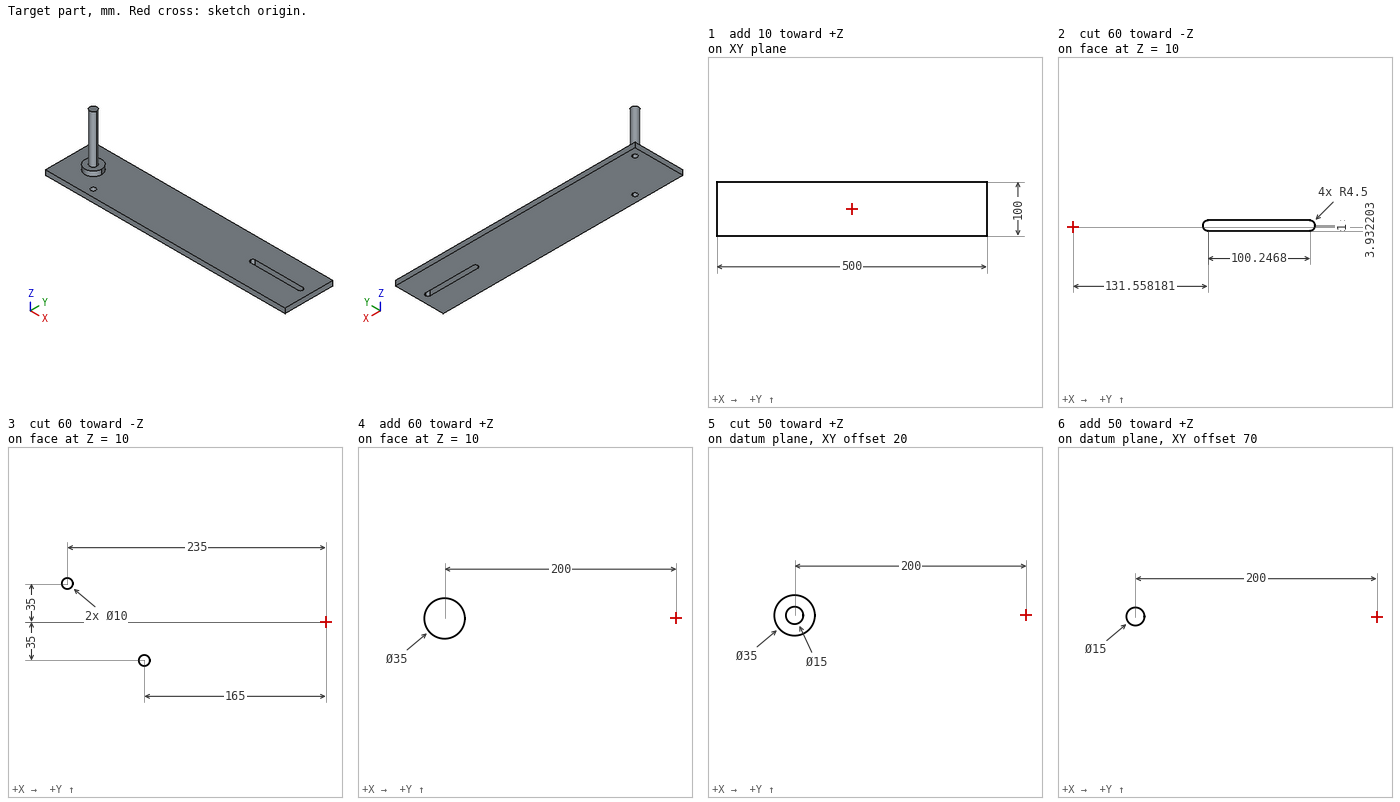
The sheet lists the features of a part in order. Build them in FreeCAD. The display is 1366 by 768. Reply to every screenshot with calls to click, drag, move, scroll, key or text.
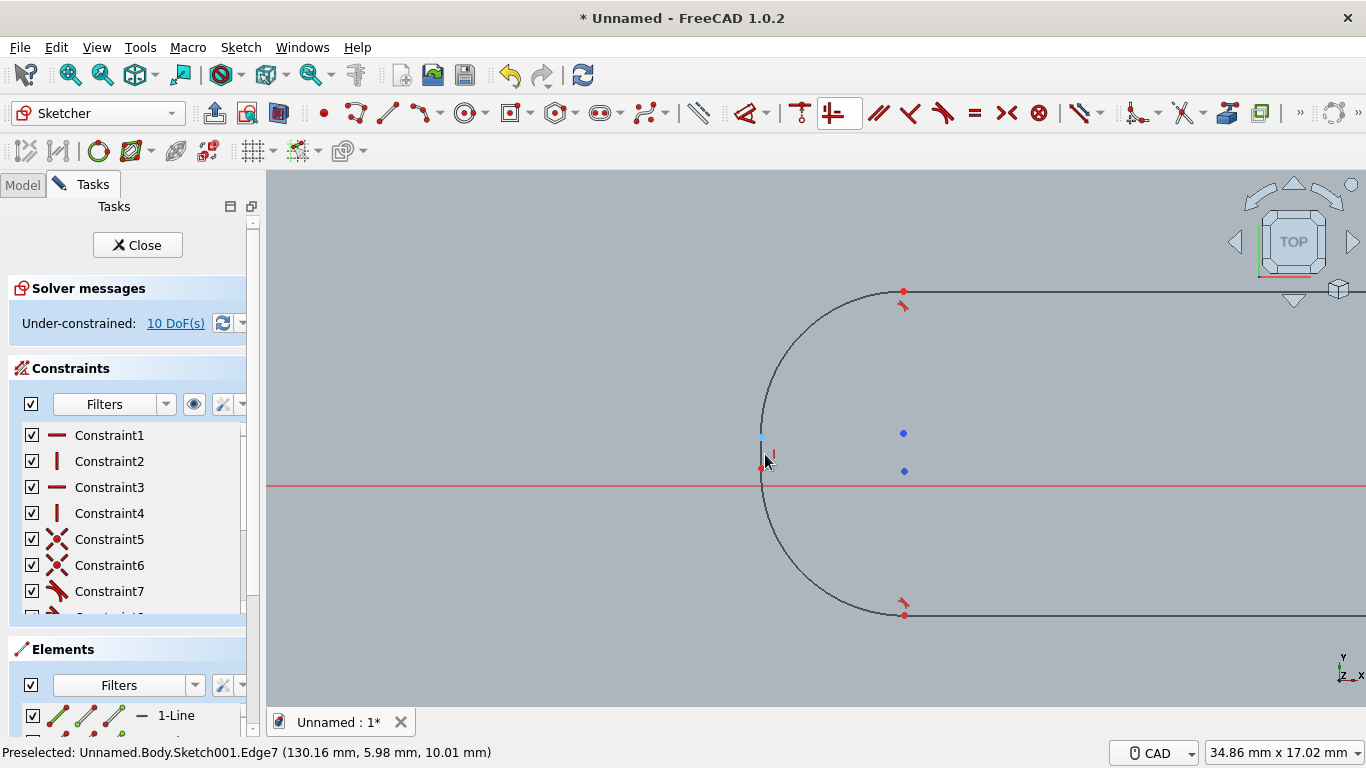
click(761, 453)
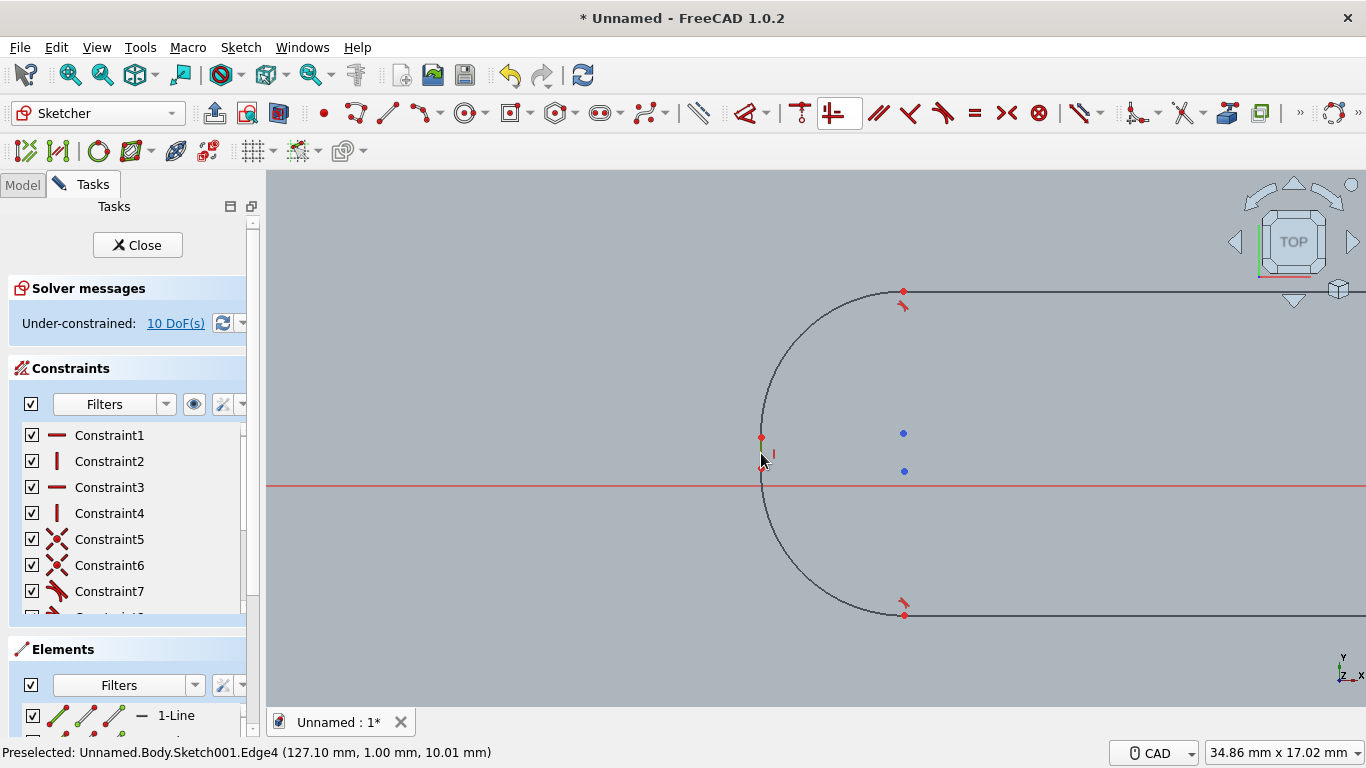
scroll(774, 437, down, 12)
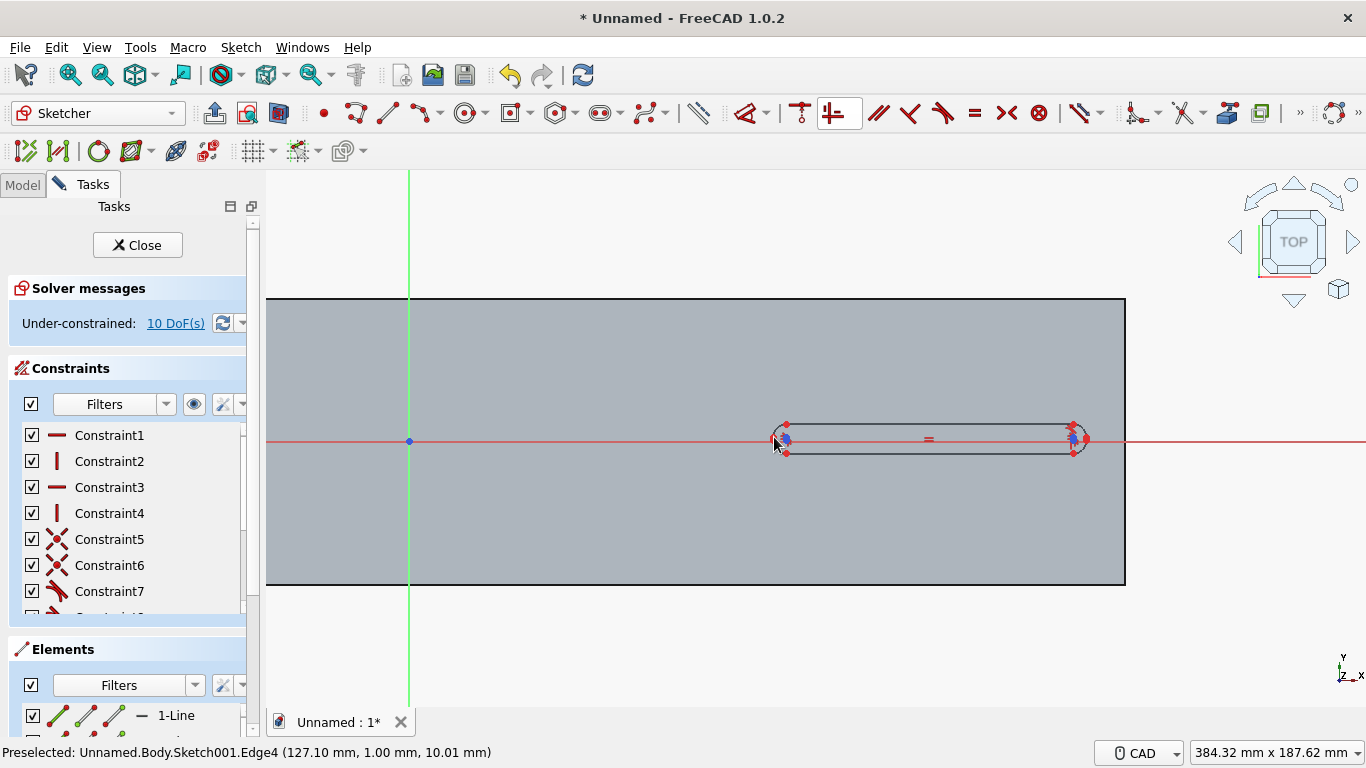
scroll(780, 426, up, 5)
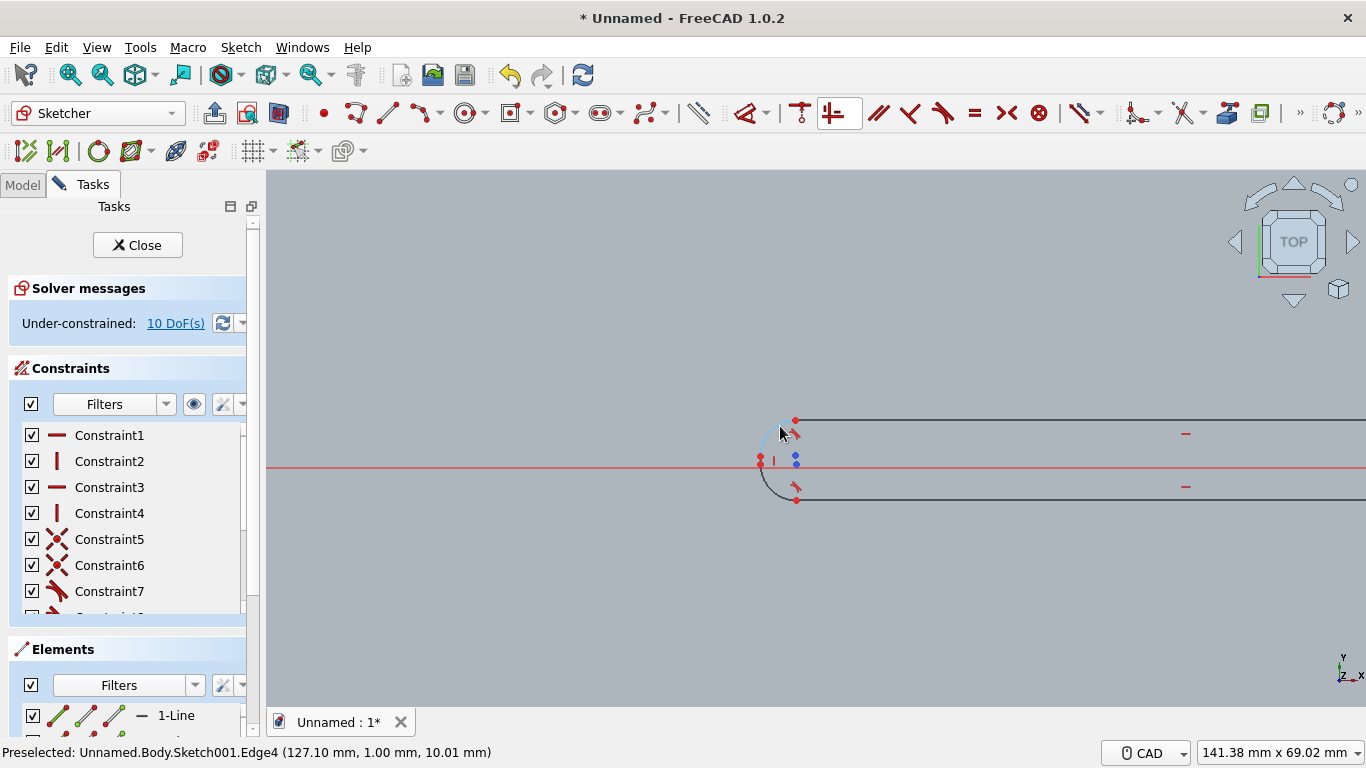
click(780, 424)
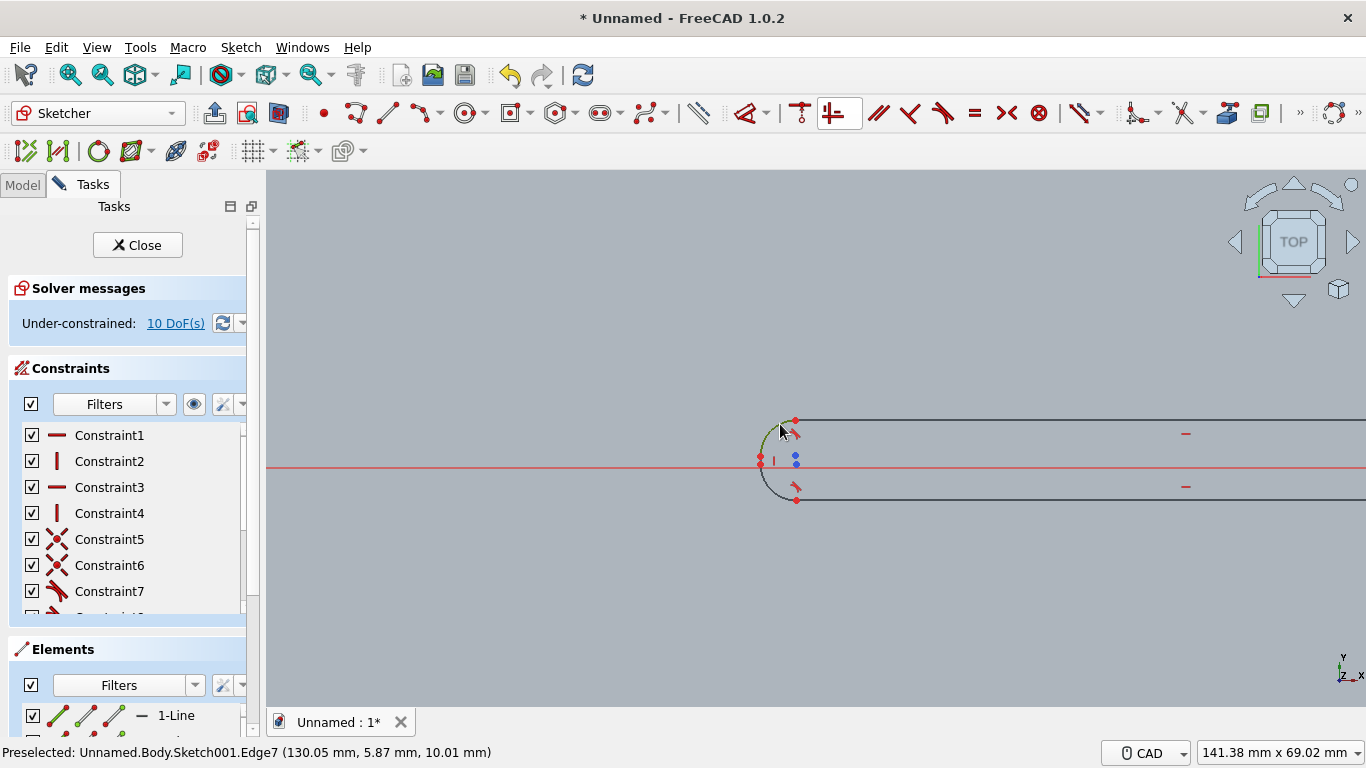
key(t)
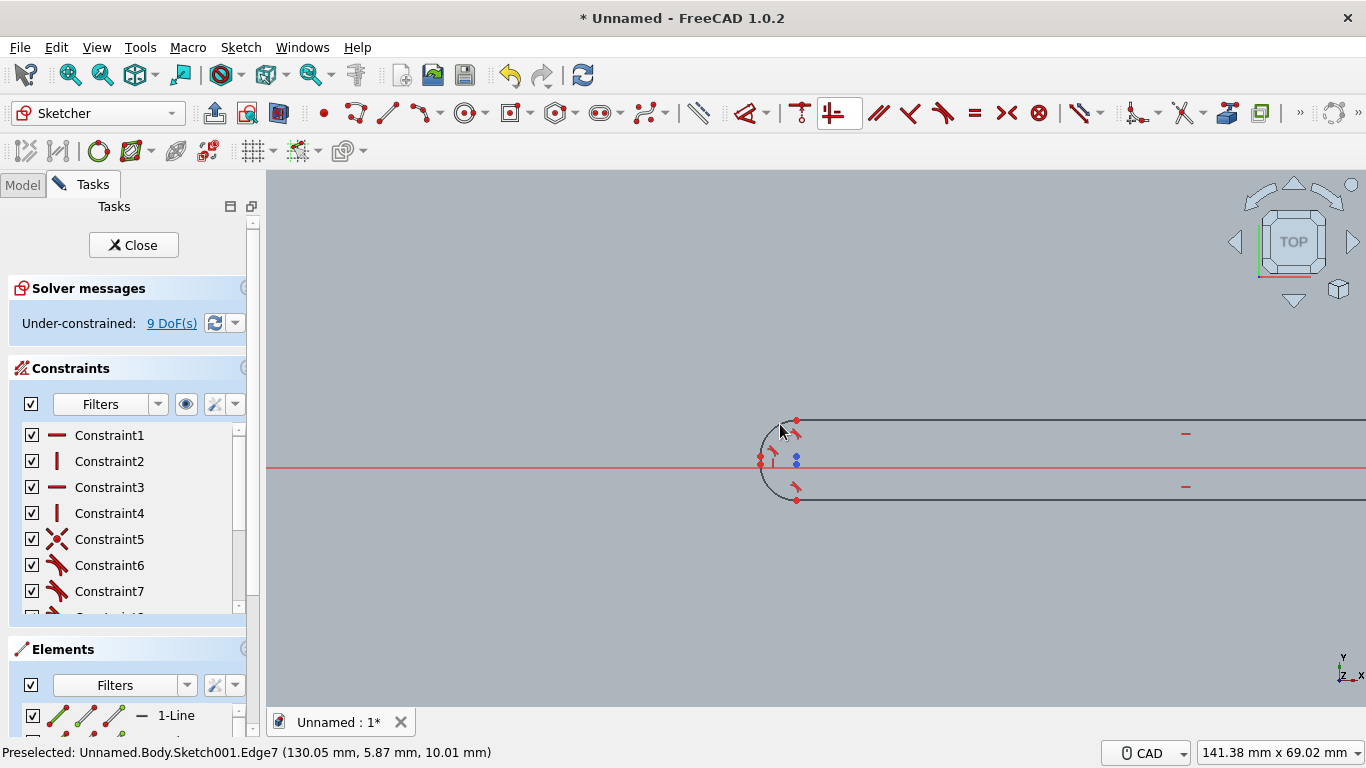
scroll(761, 460, up, 7)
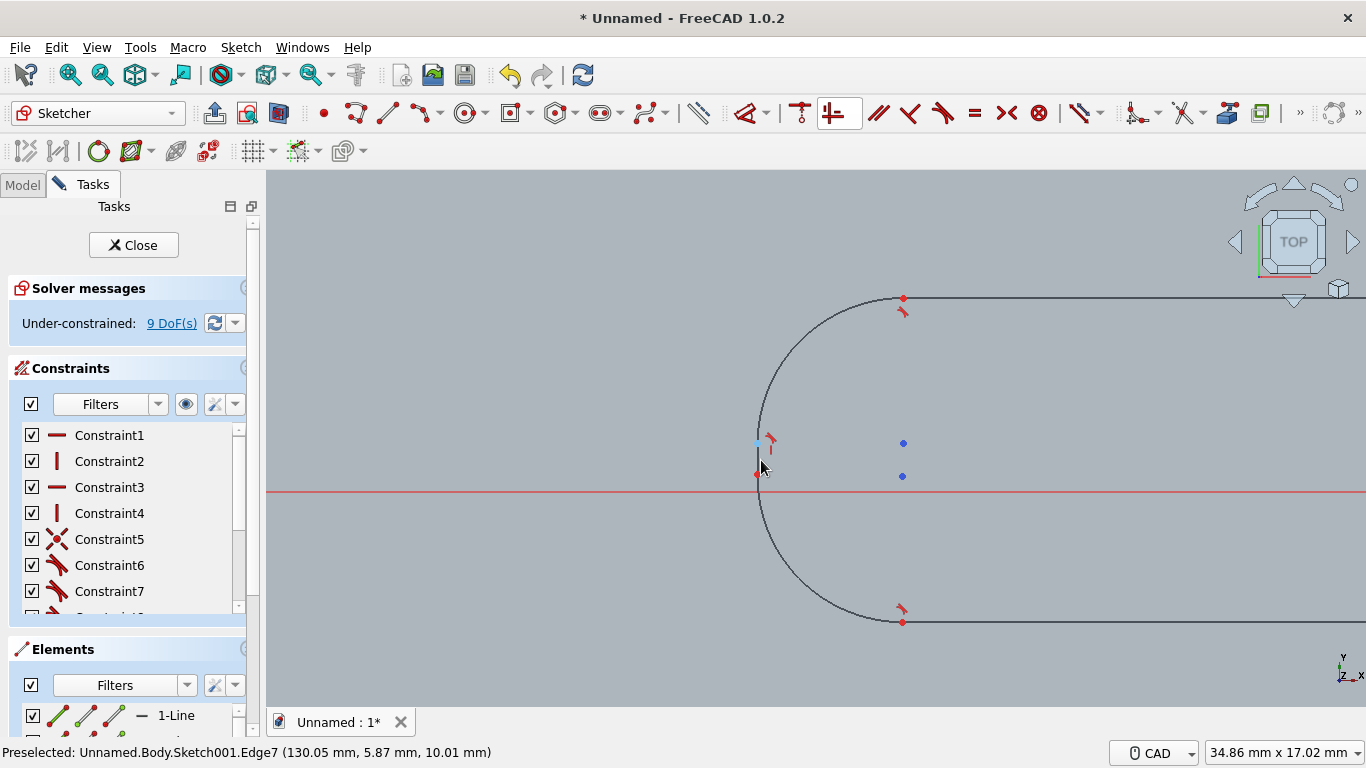
click(758, 459)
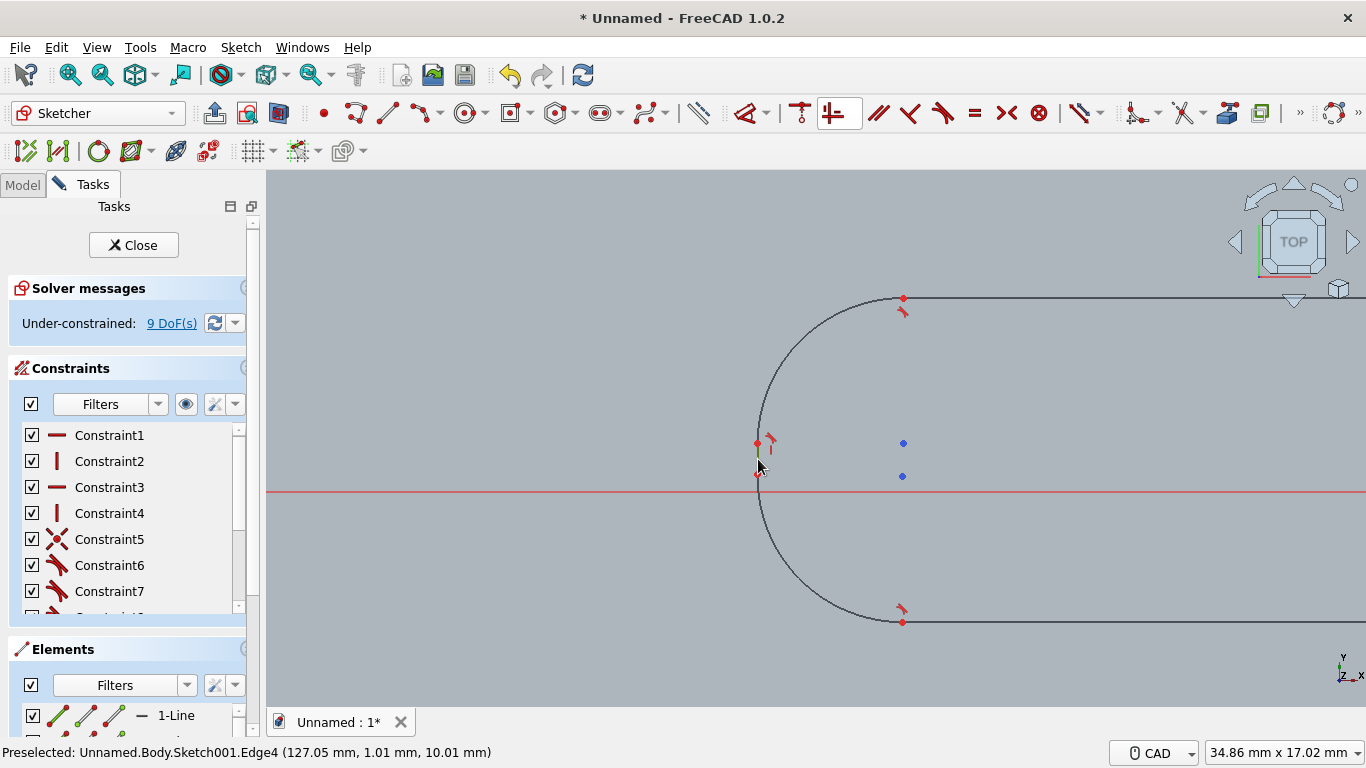
scroll(775, 437, down, 12)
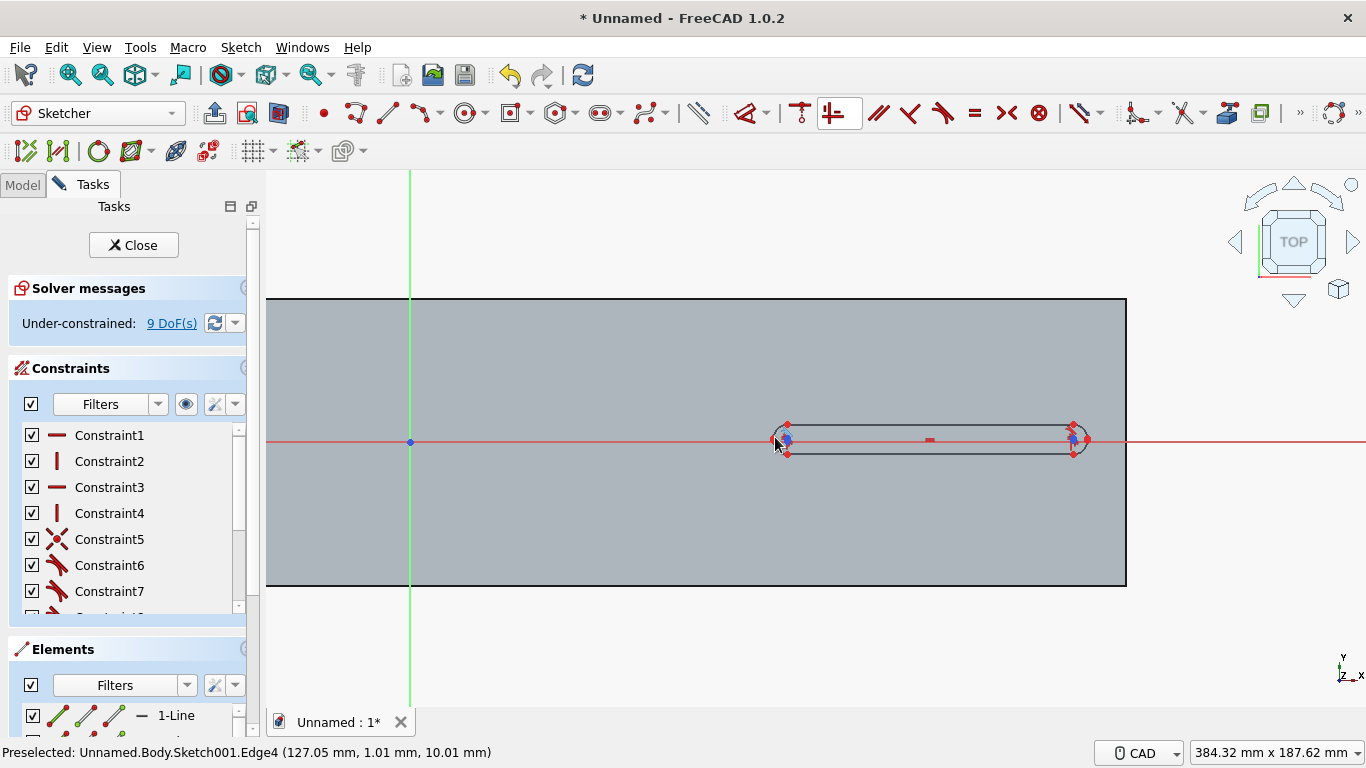
scroll(775, 447, up, 6)